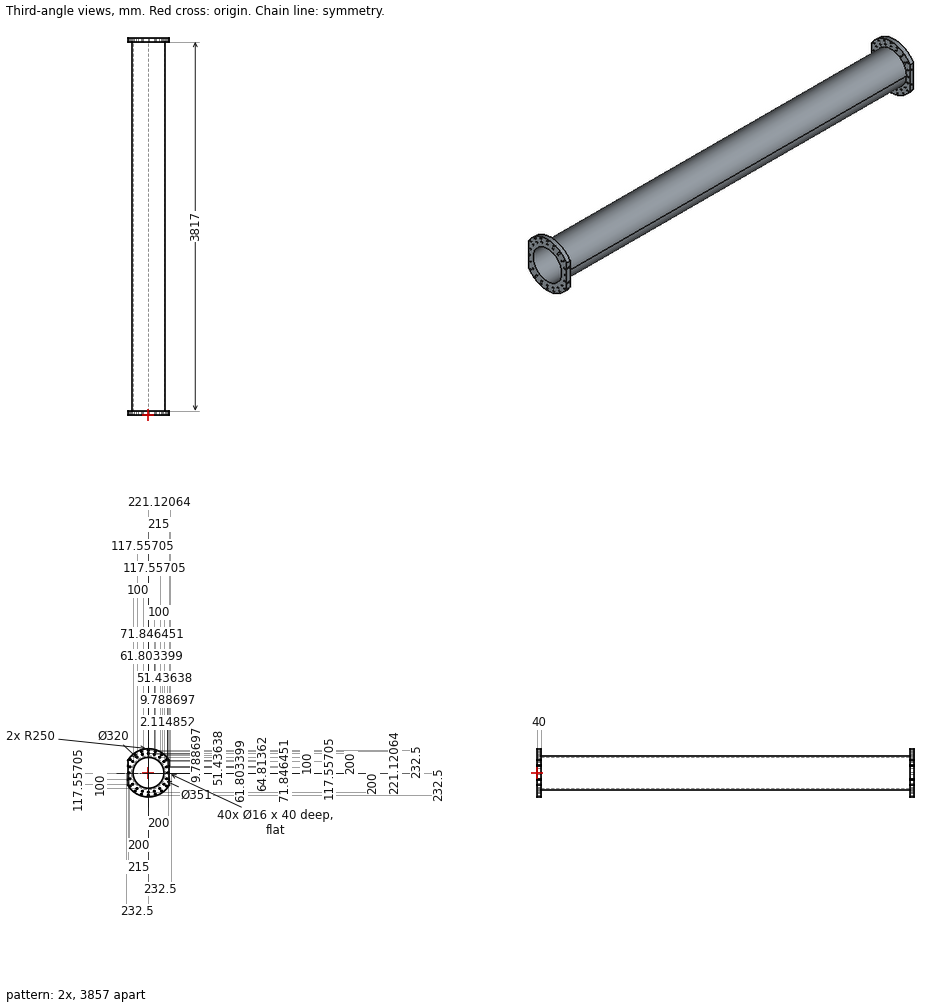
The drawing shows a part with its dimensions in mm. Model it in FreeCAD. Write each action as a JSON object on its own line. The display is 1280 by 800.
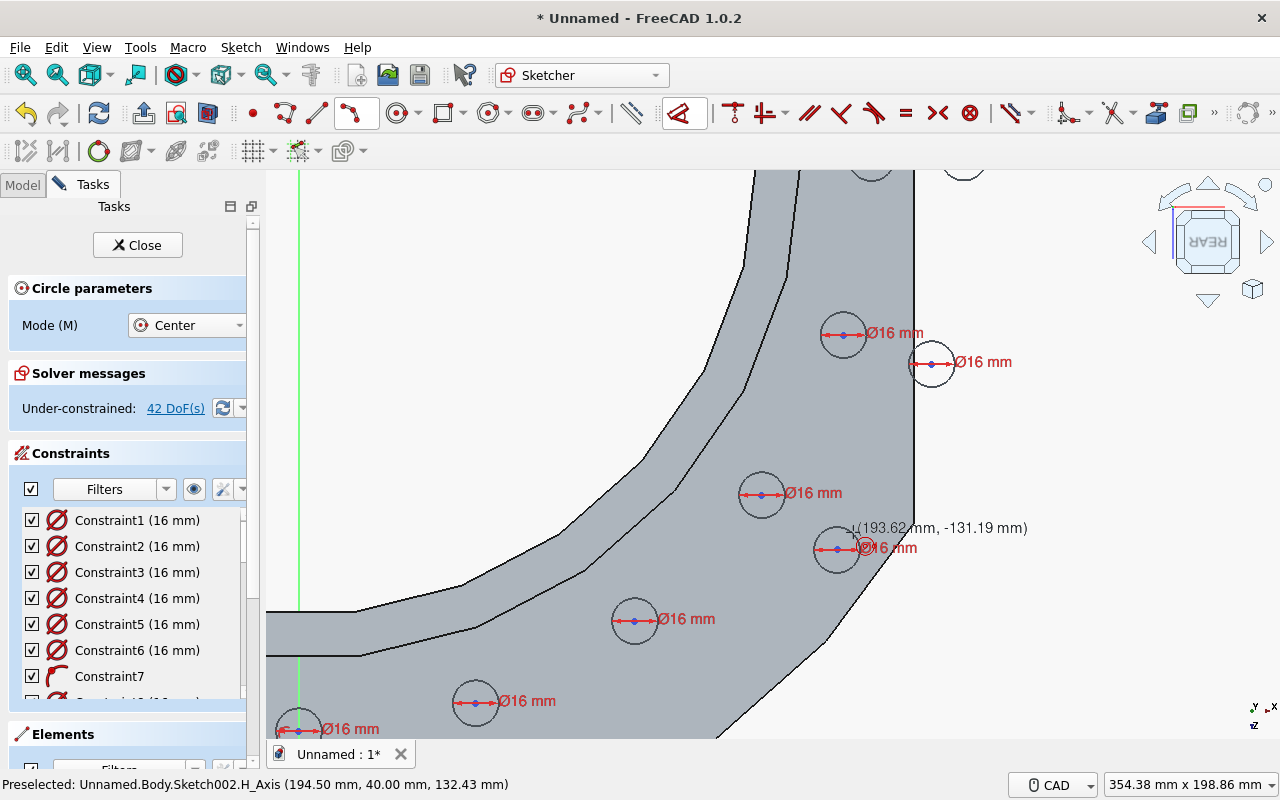
{"action": "left_click", "coordinate": [690, 696]}
{"action": "mouse_move", "coordinate": [706, 680]}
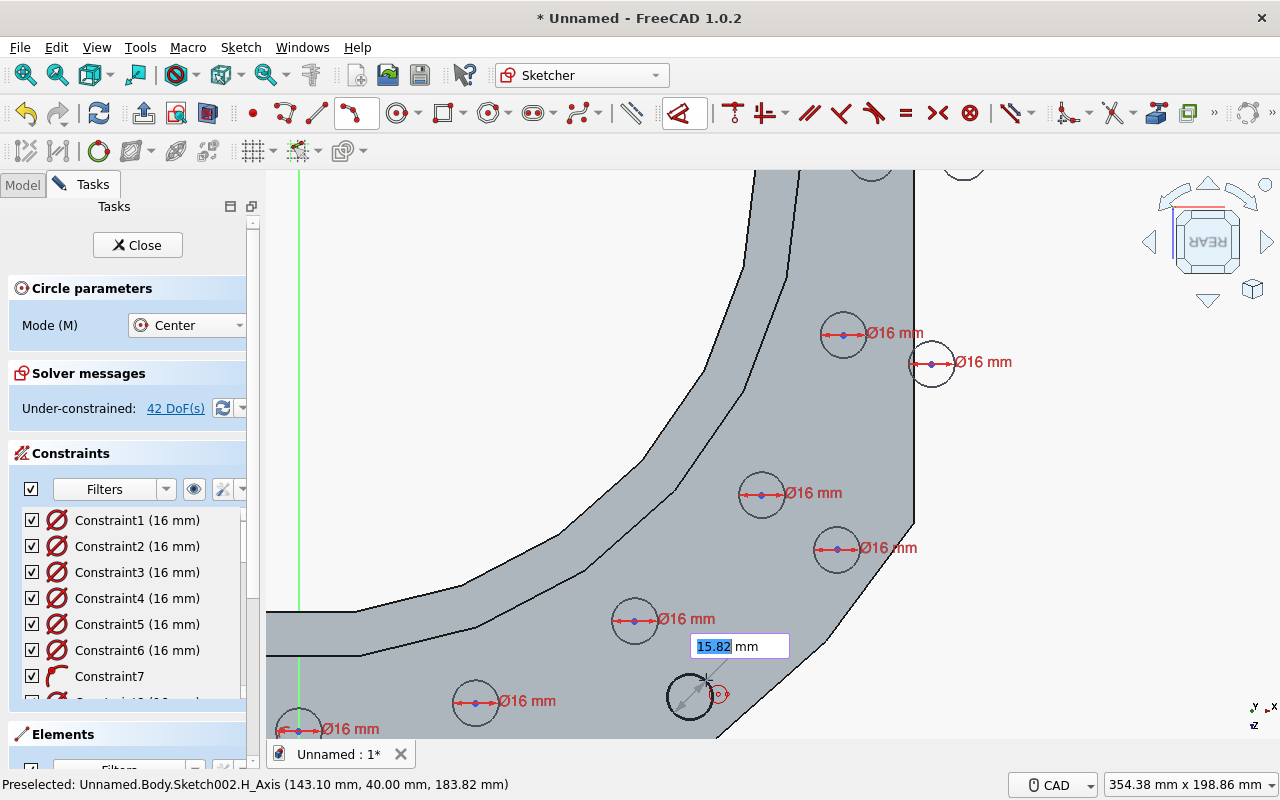
{"action": "type", "text": "16"}
{"action": "key", "text": "Return"}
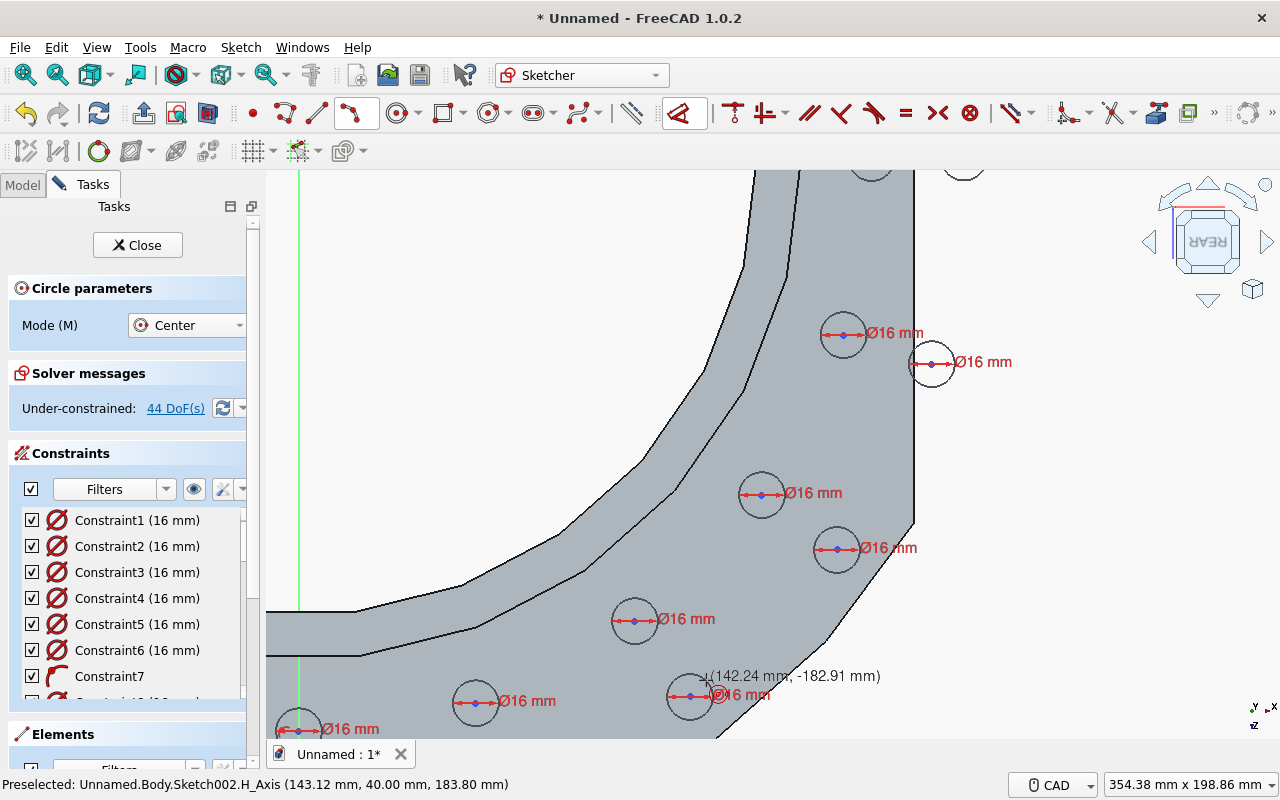
{"action": "scroll", "coordinate": [837, 552], "scroll_direction": "down", "scroll_amount": 7}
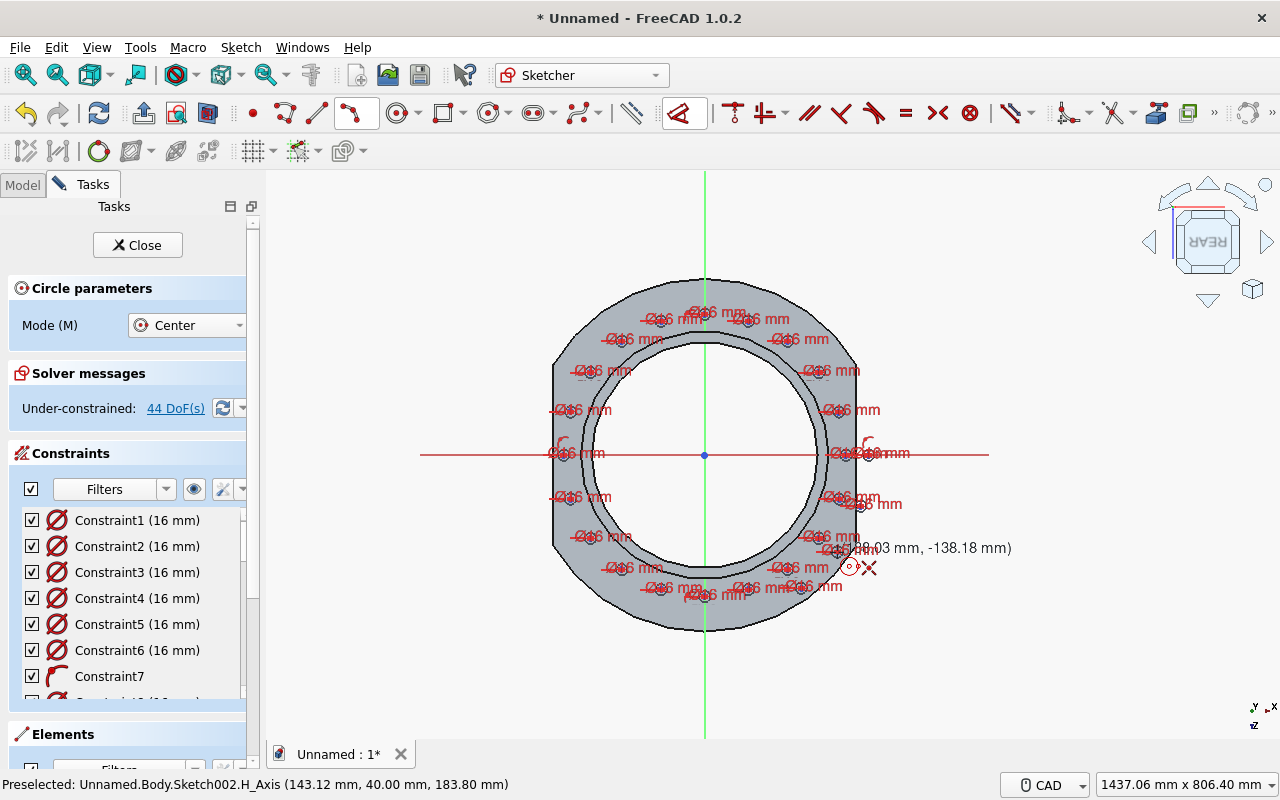
{"action": "scroll", "coordinate": [755, 611], "scroll_direction": "up", "scroll_amount": 7}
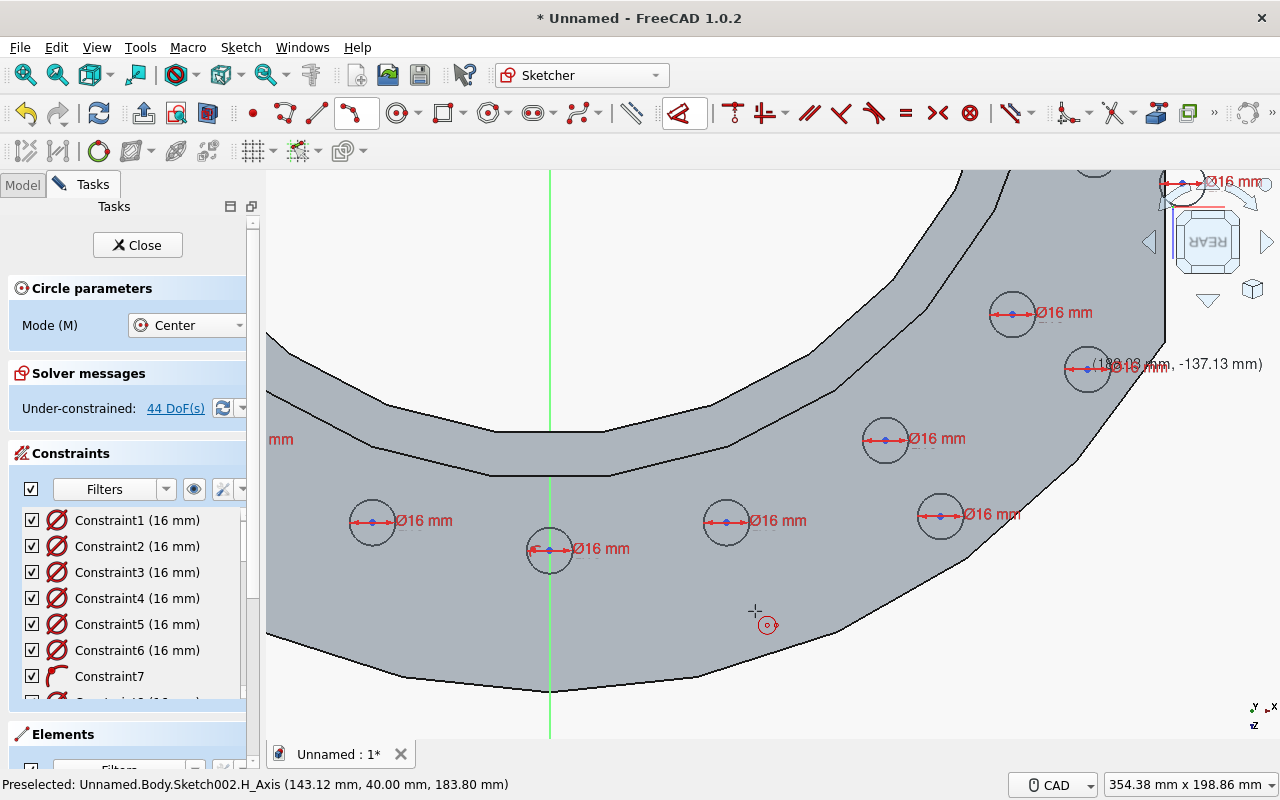
{"action": "left_click", "coordinate": [755, 610]}
{"action": "mouse_move", "coordinate": [772, 594]}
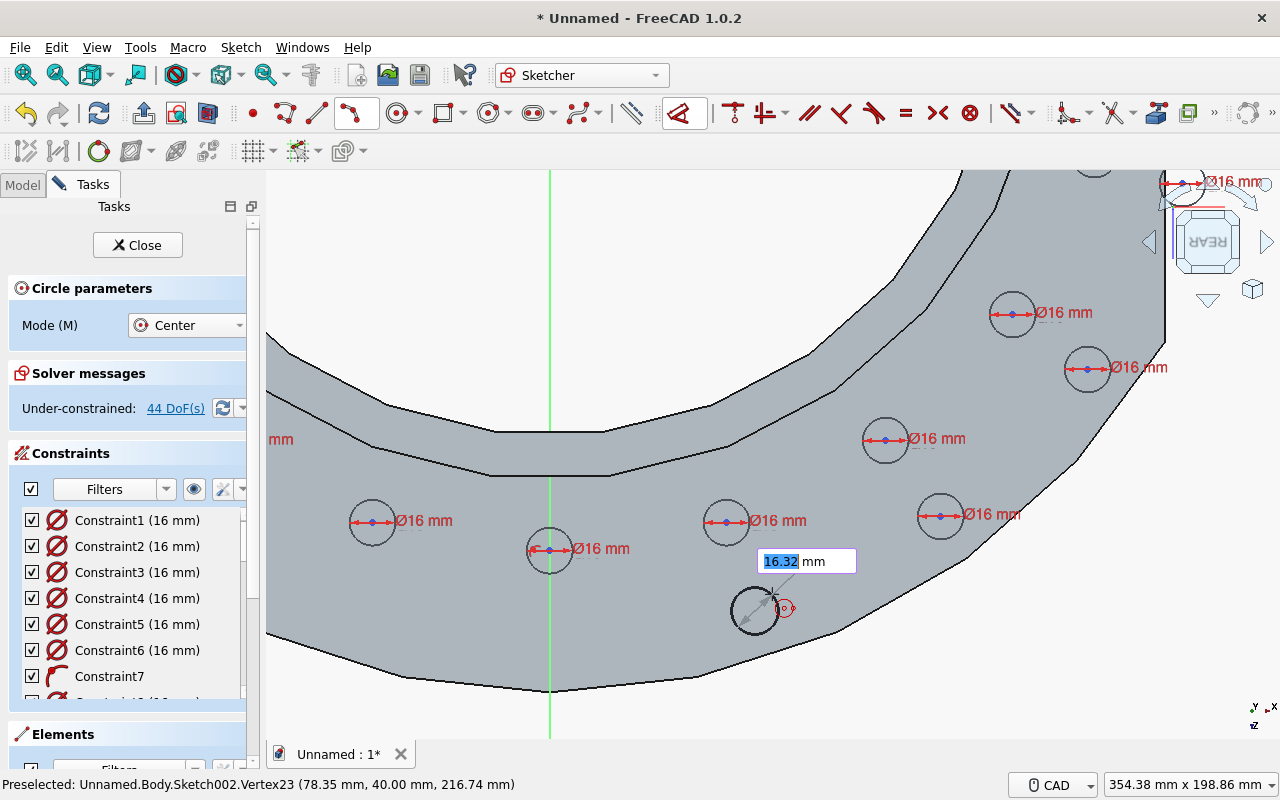
{"action": "type", "text": "16"}
{"action": "key", "text": "Return"}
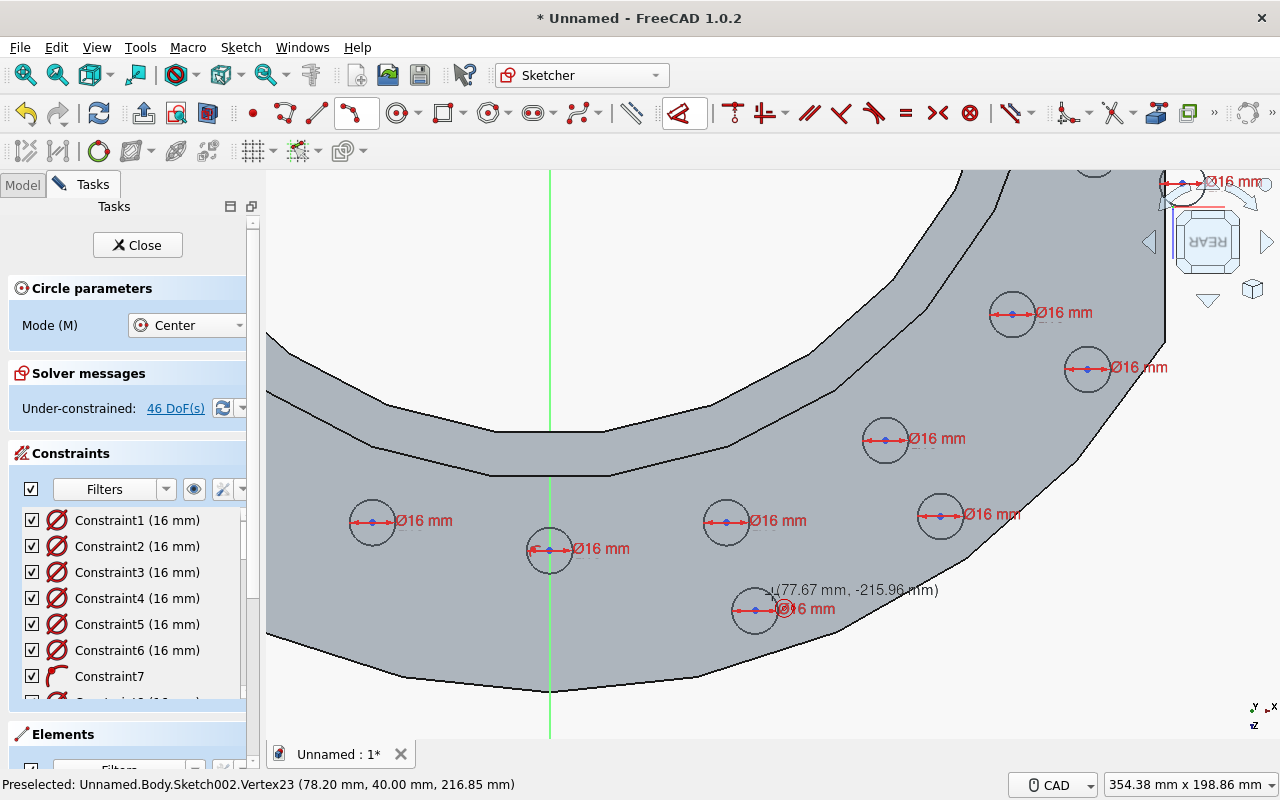
{"action": "left_click", "coordinate": [550, 642]}
{"action": "mouse_move", "coordinate": [566, 626]}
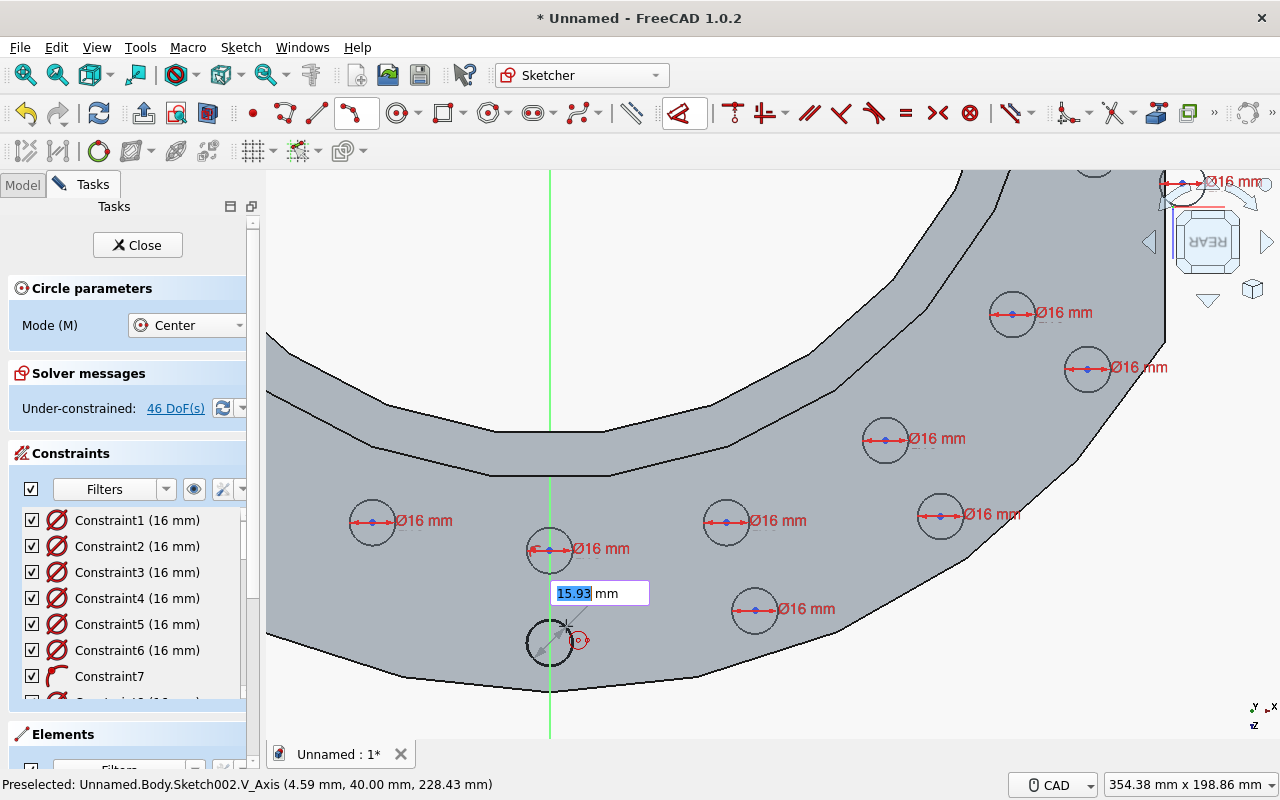
{"action": "type", "text": "16"}
{"action": "key", "text": "Return"}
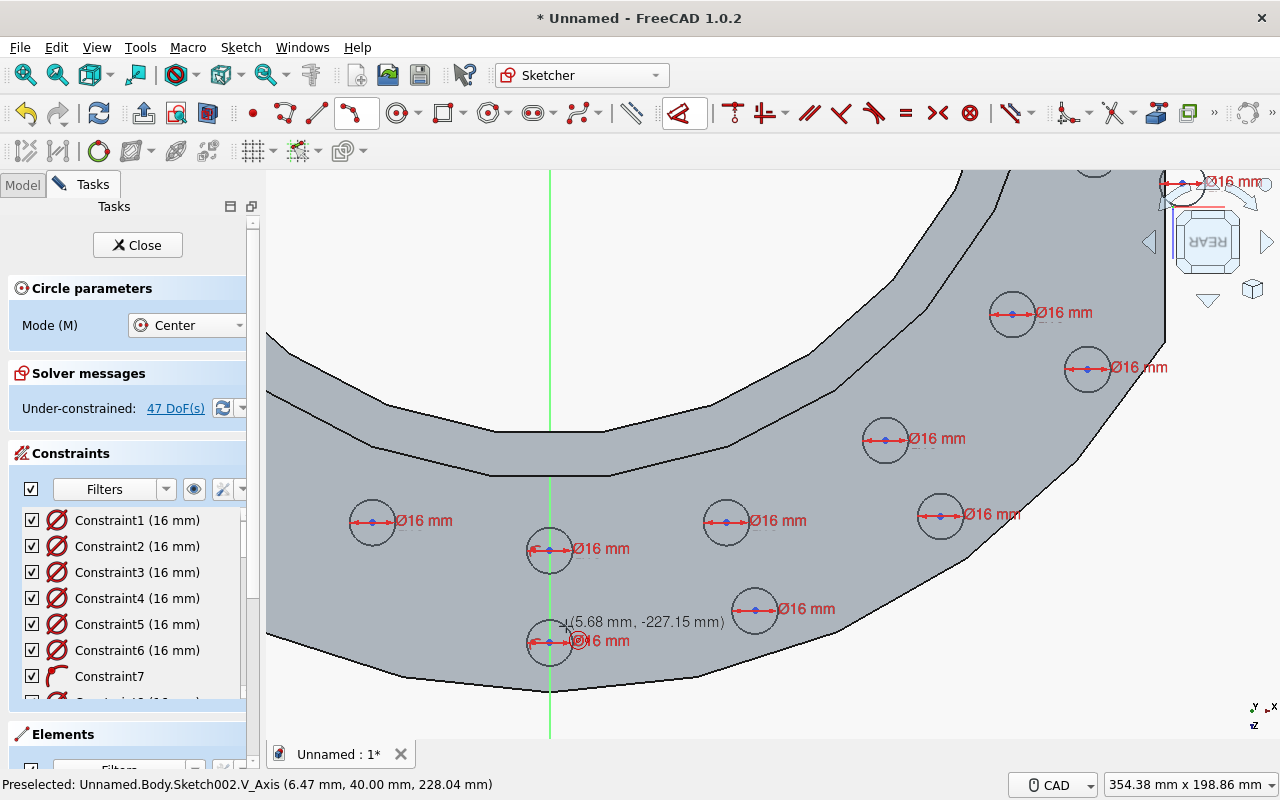
{"action": "left_click", "coordinate": [344, 610]}
{"action": "mouse_move", "coordinate": [360, 594]}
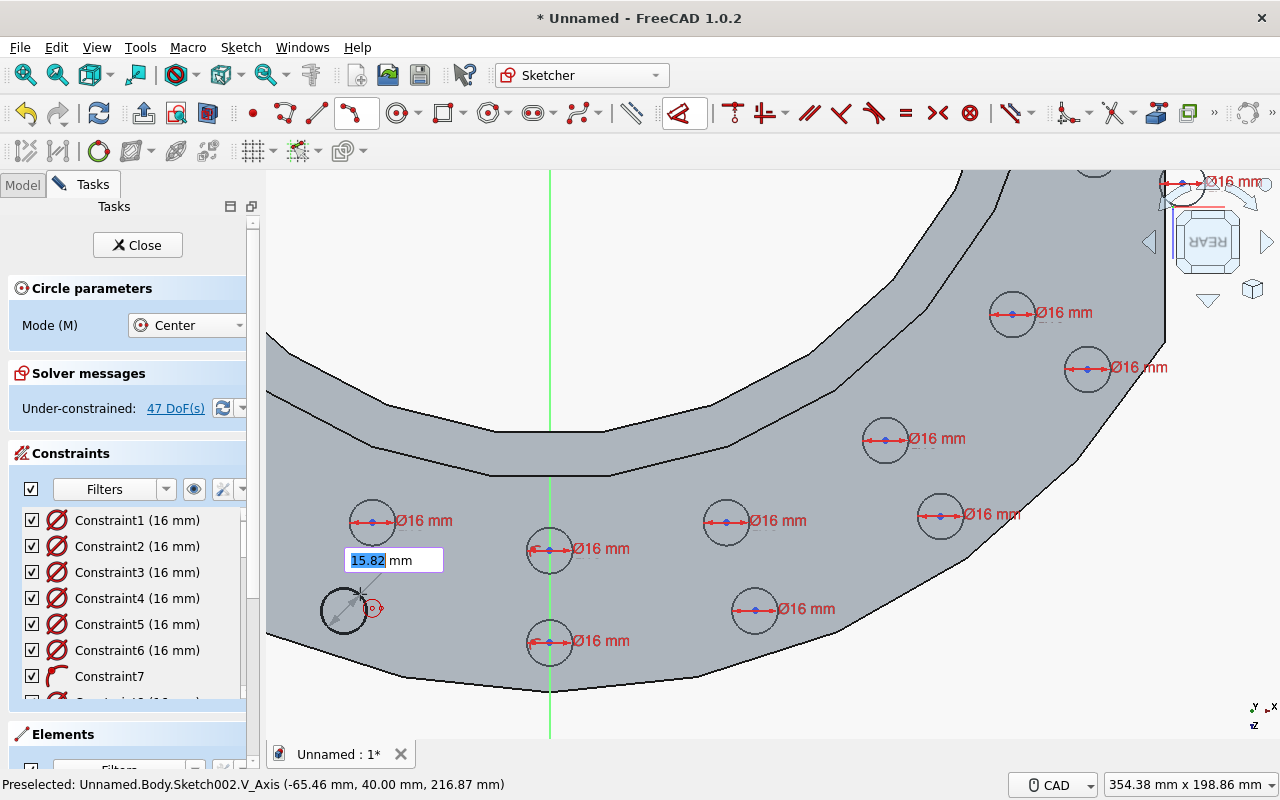
{"action": "type", "text": "16"}
{"action": "key", "text": "Return"}